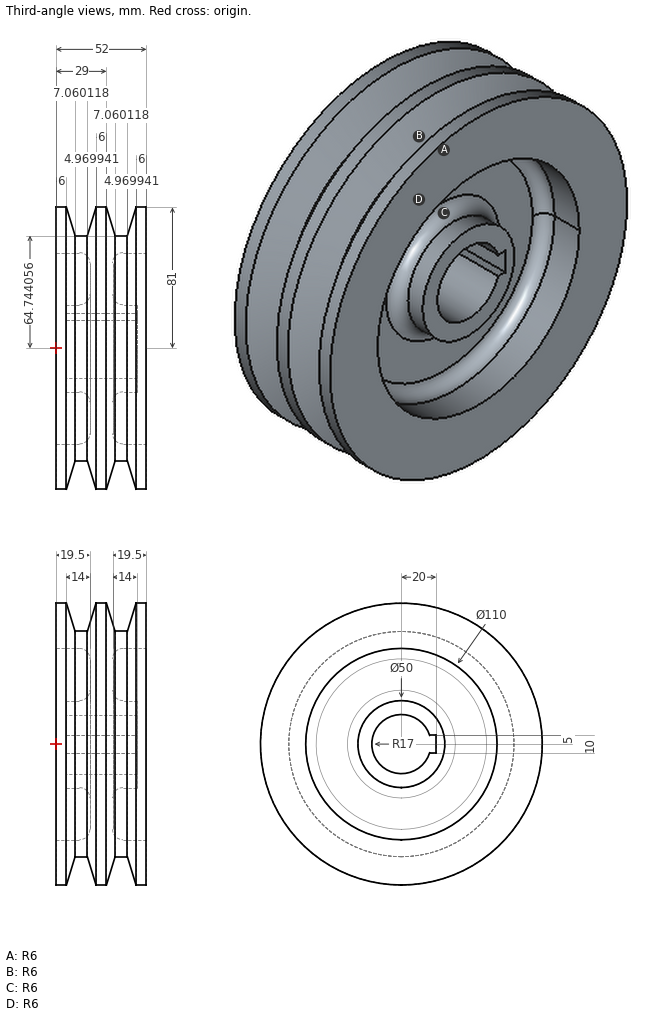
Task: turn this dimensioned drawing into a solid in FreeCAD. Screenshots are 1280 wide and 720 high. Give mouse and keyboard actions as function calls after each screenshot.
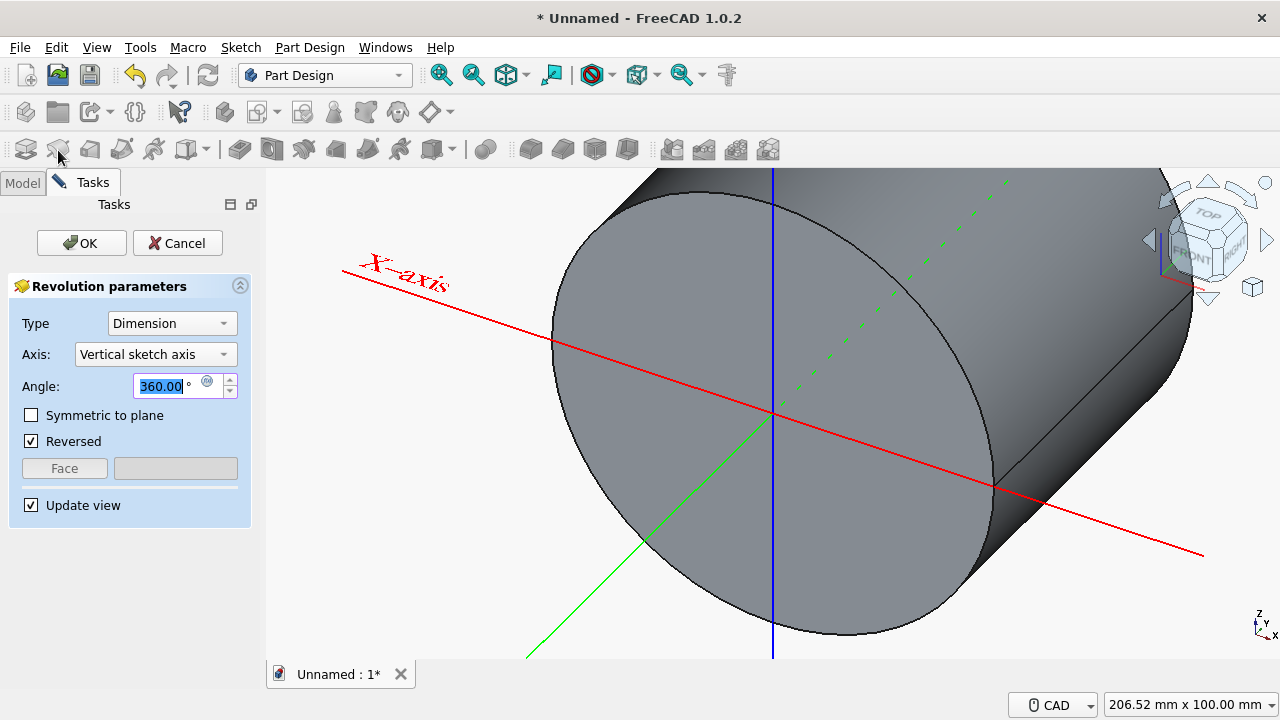
click(156, 354)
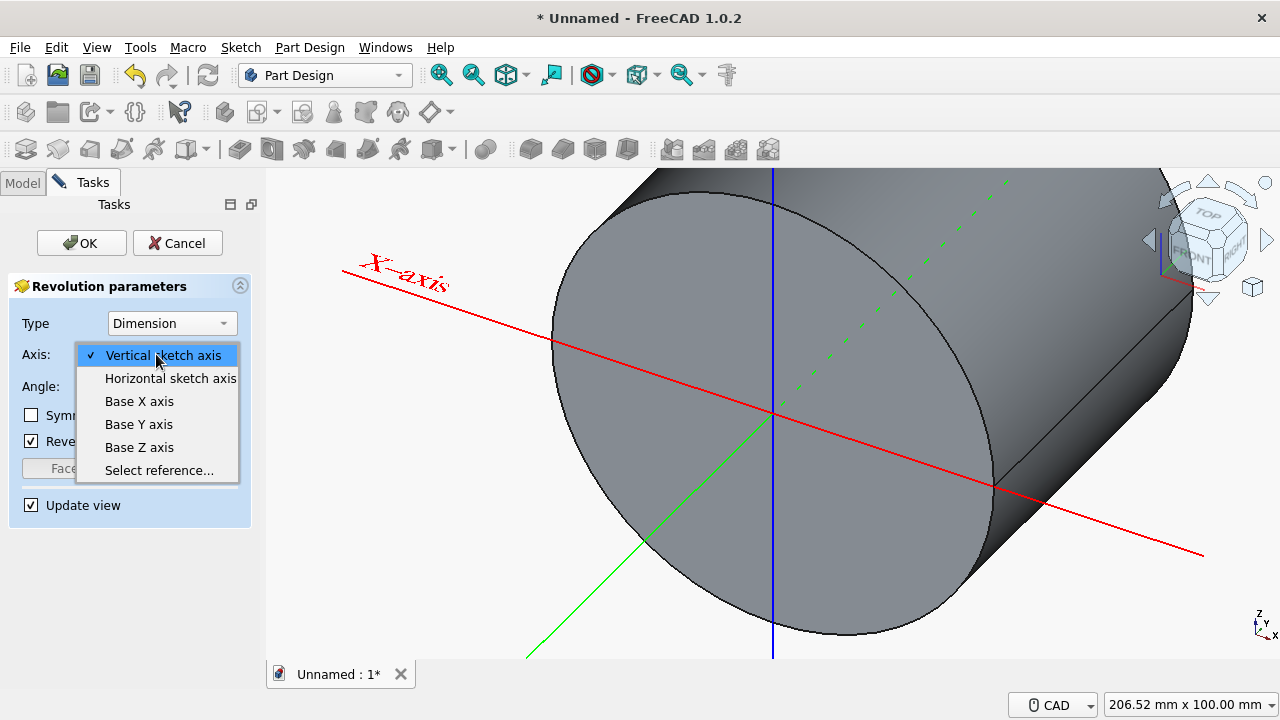
click(156, 378)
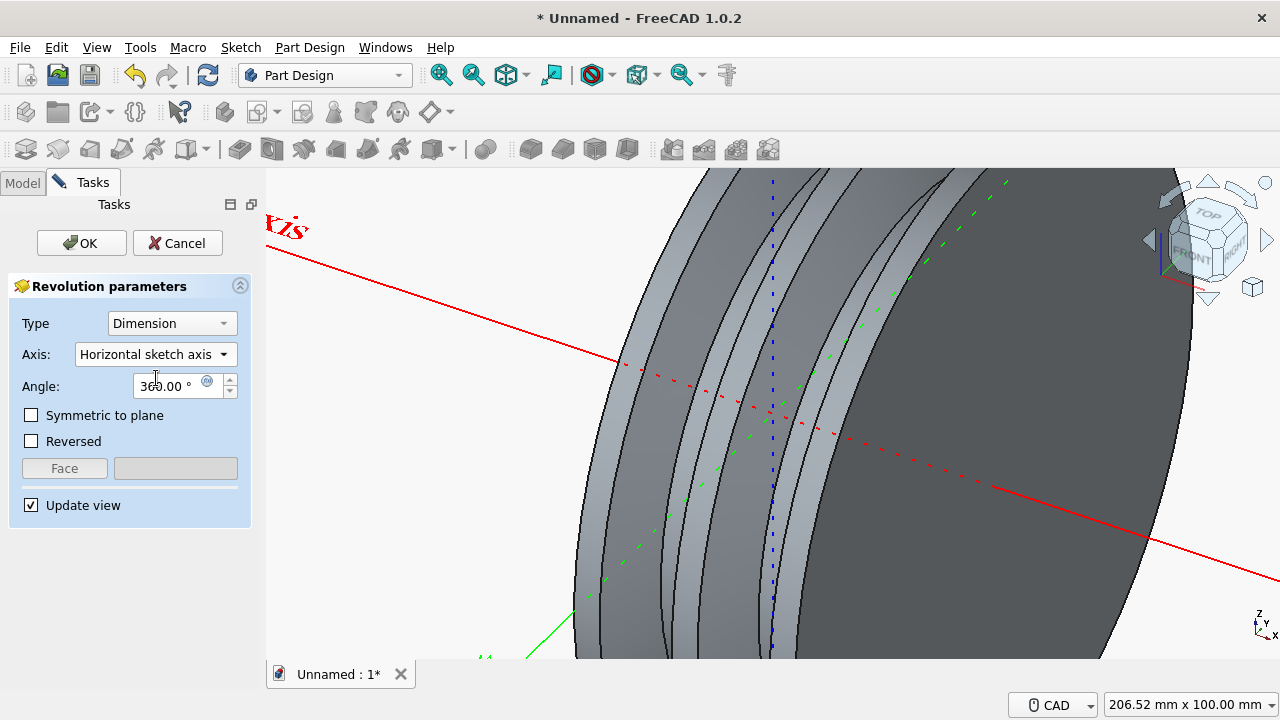
click(82, 243)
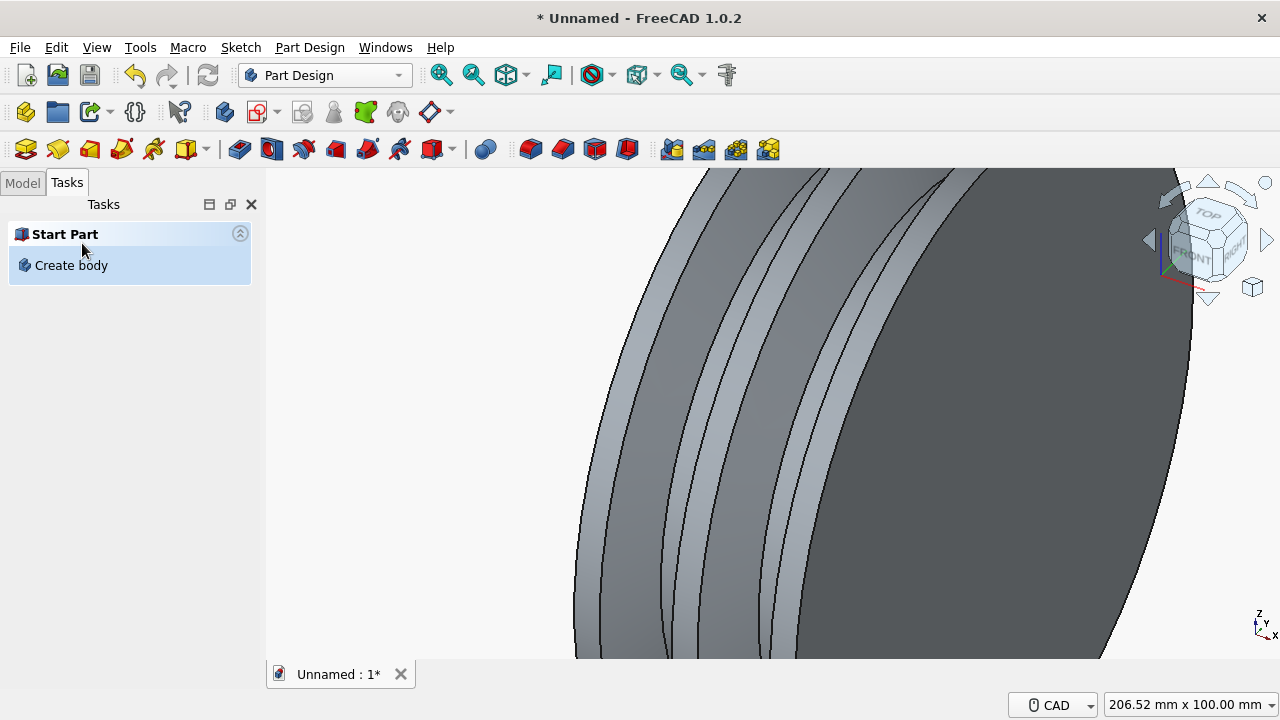
click(442, 76)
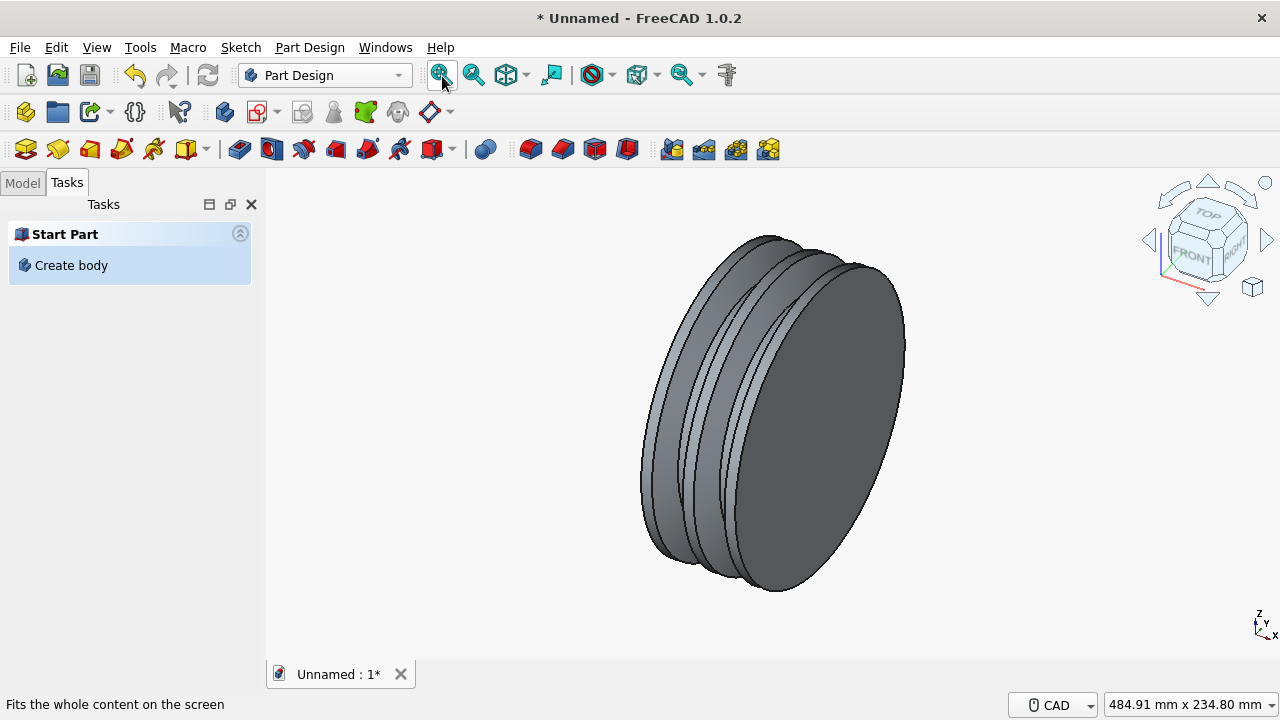
click(820, 428)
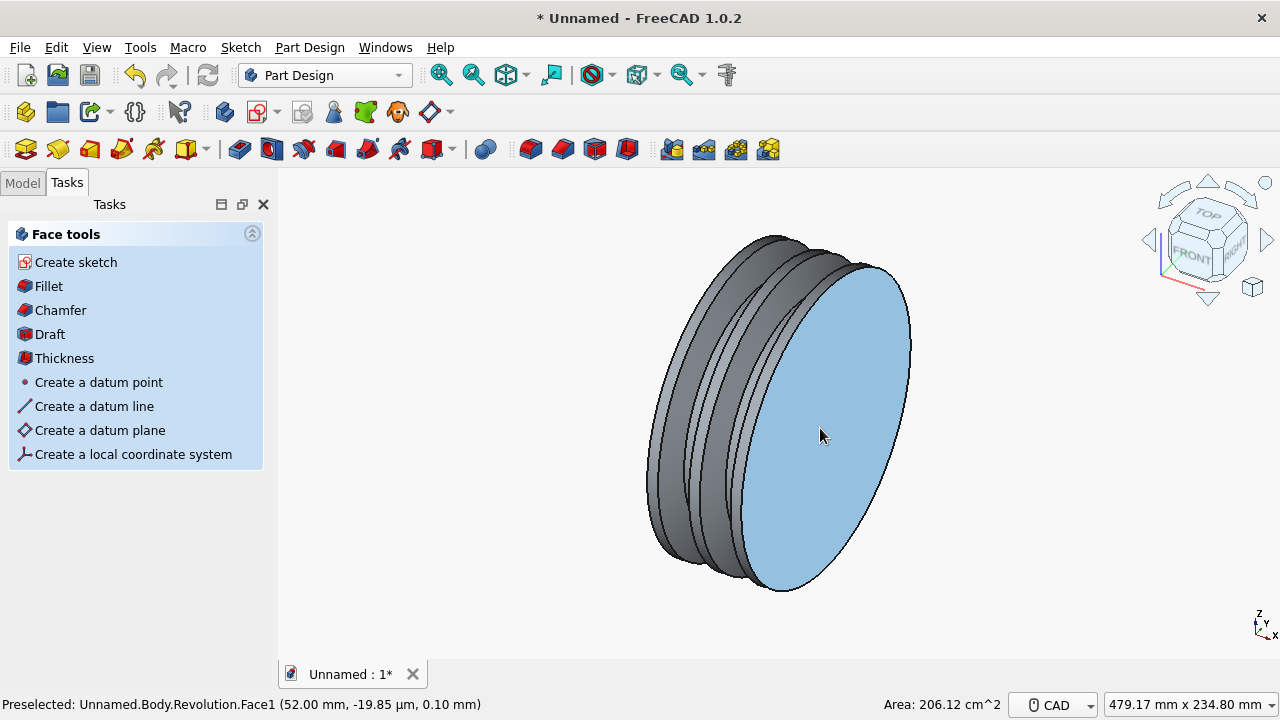
click(258, 112)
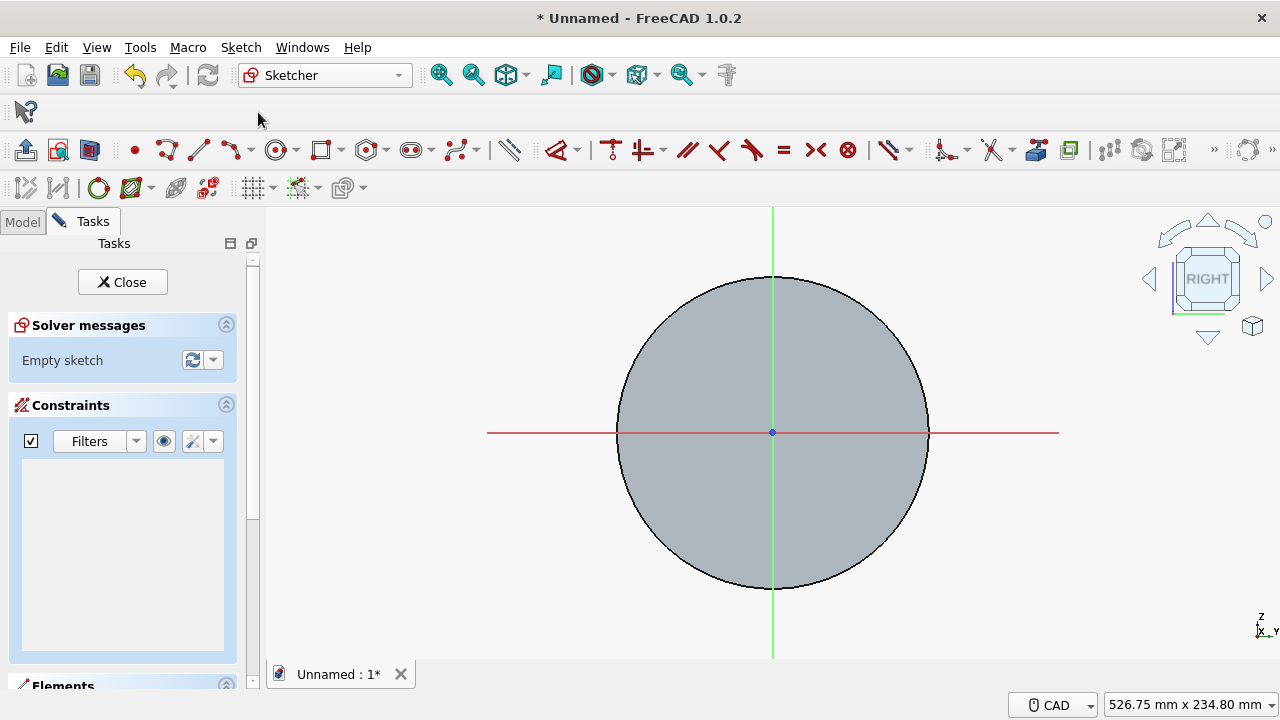
key(g)
key(c)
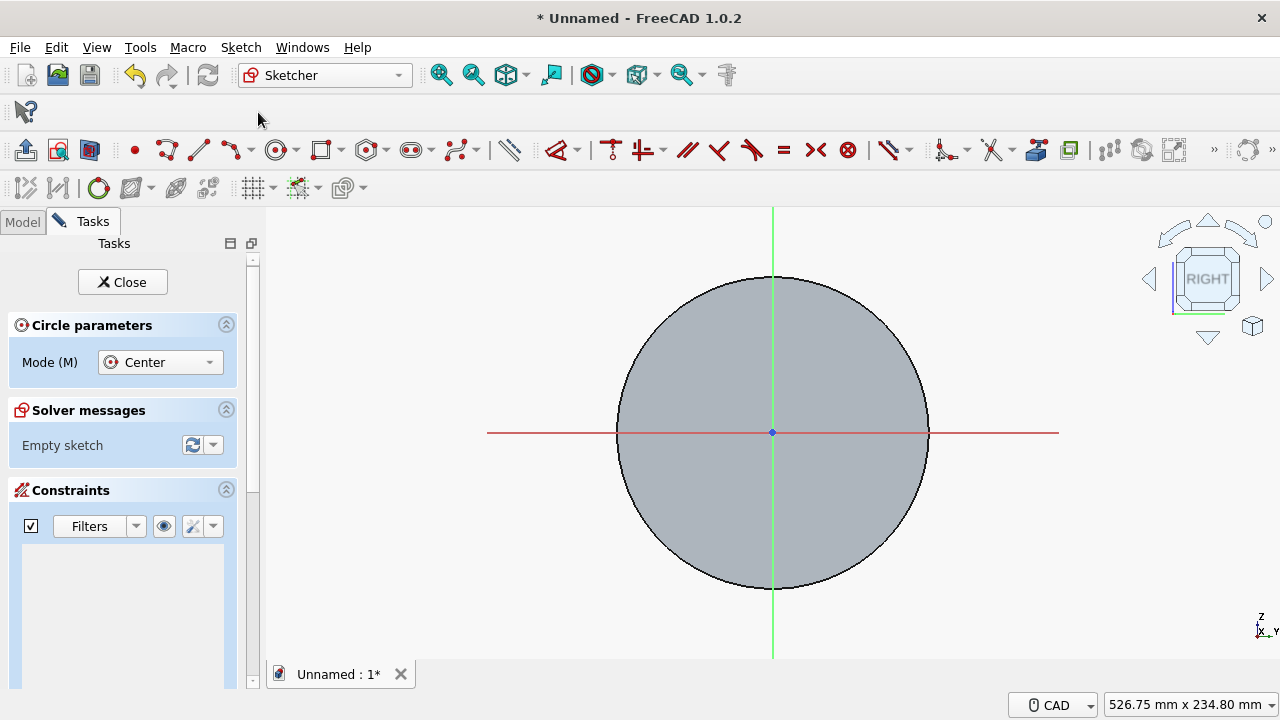
click(773, 433)
click(848, 358)
key(Escape)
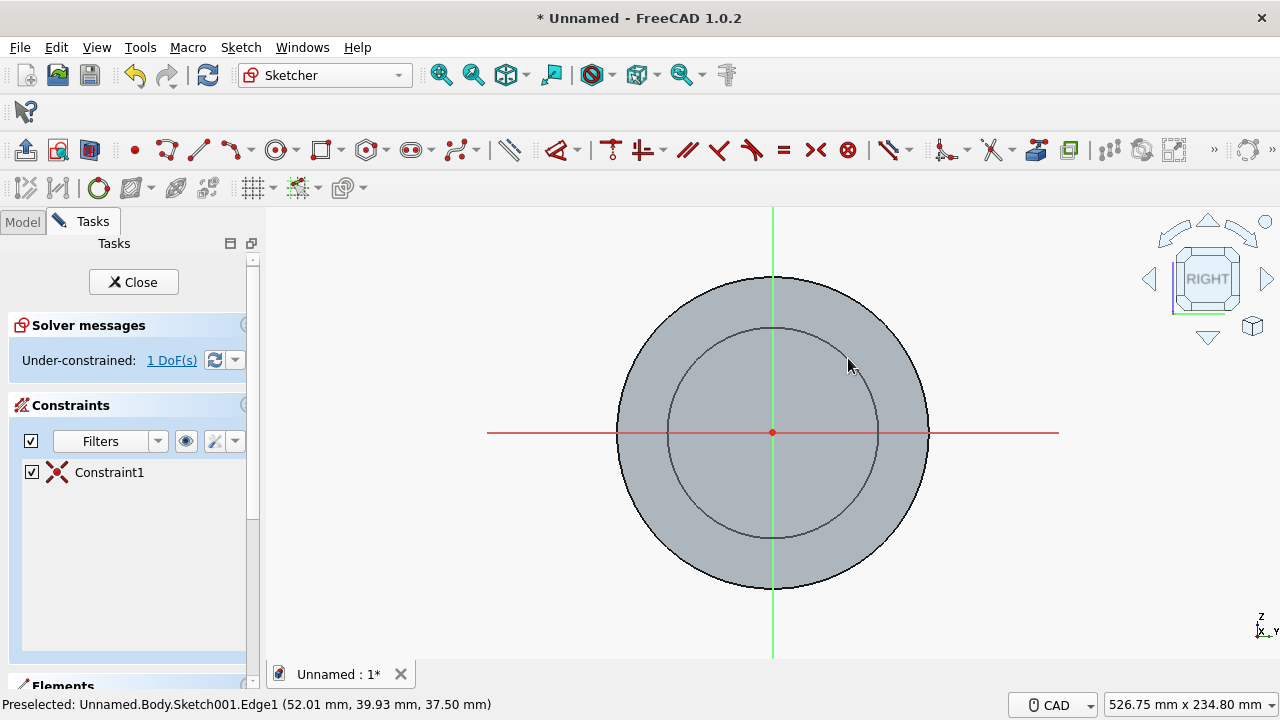
key(d)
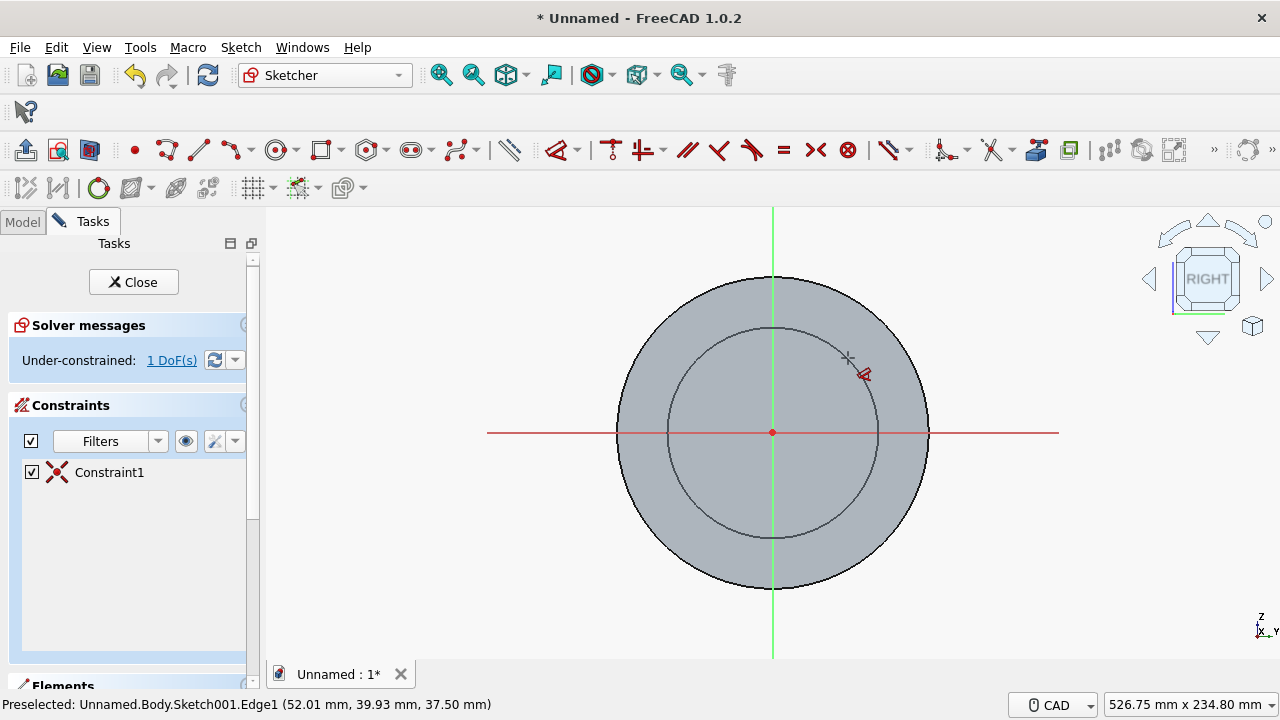
click(847, 358)
click(869, 335)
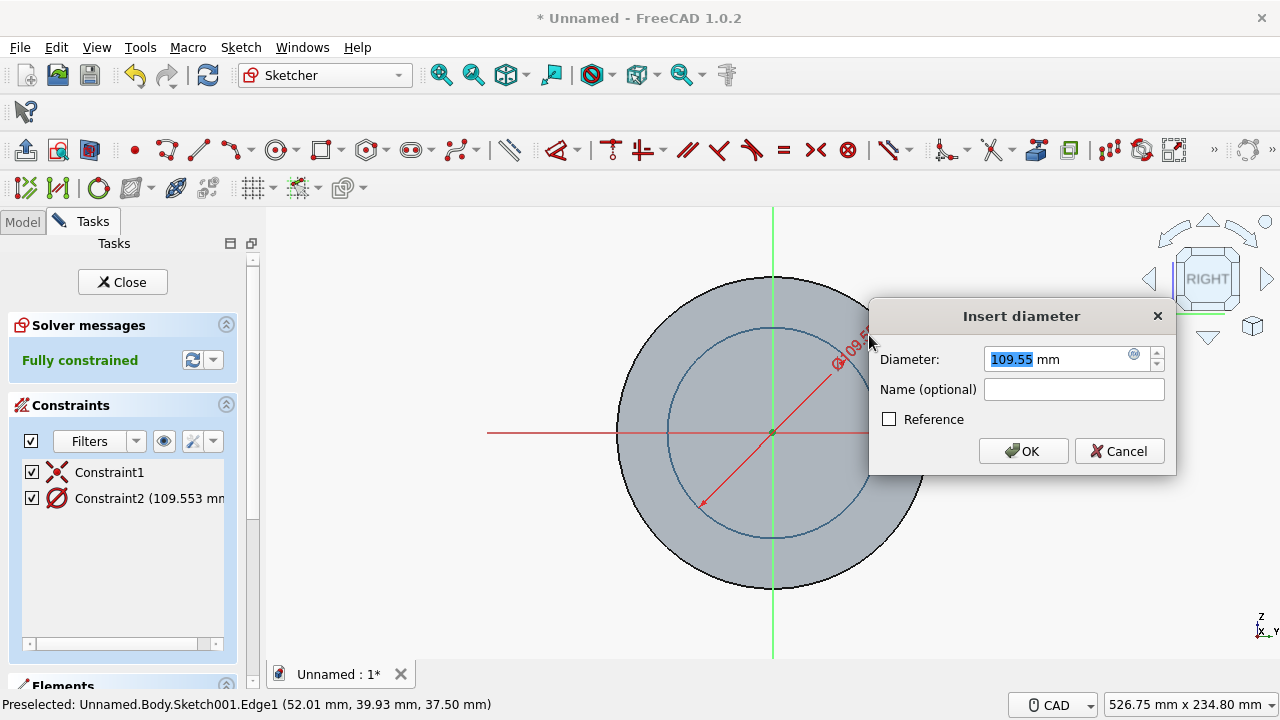
text(110)
key(Return)
key(Escape)